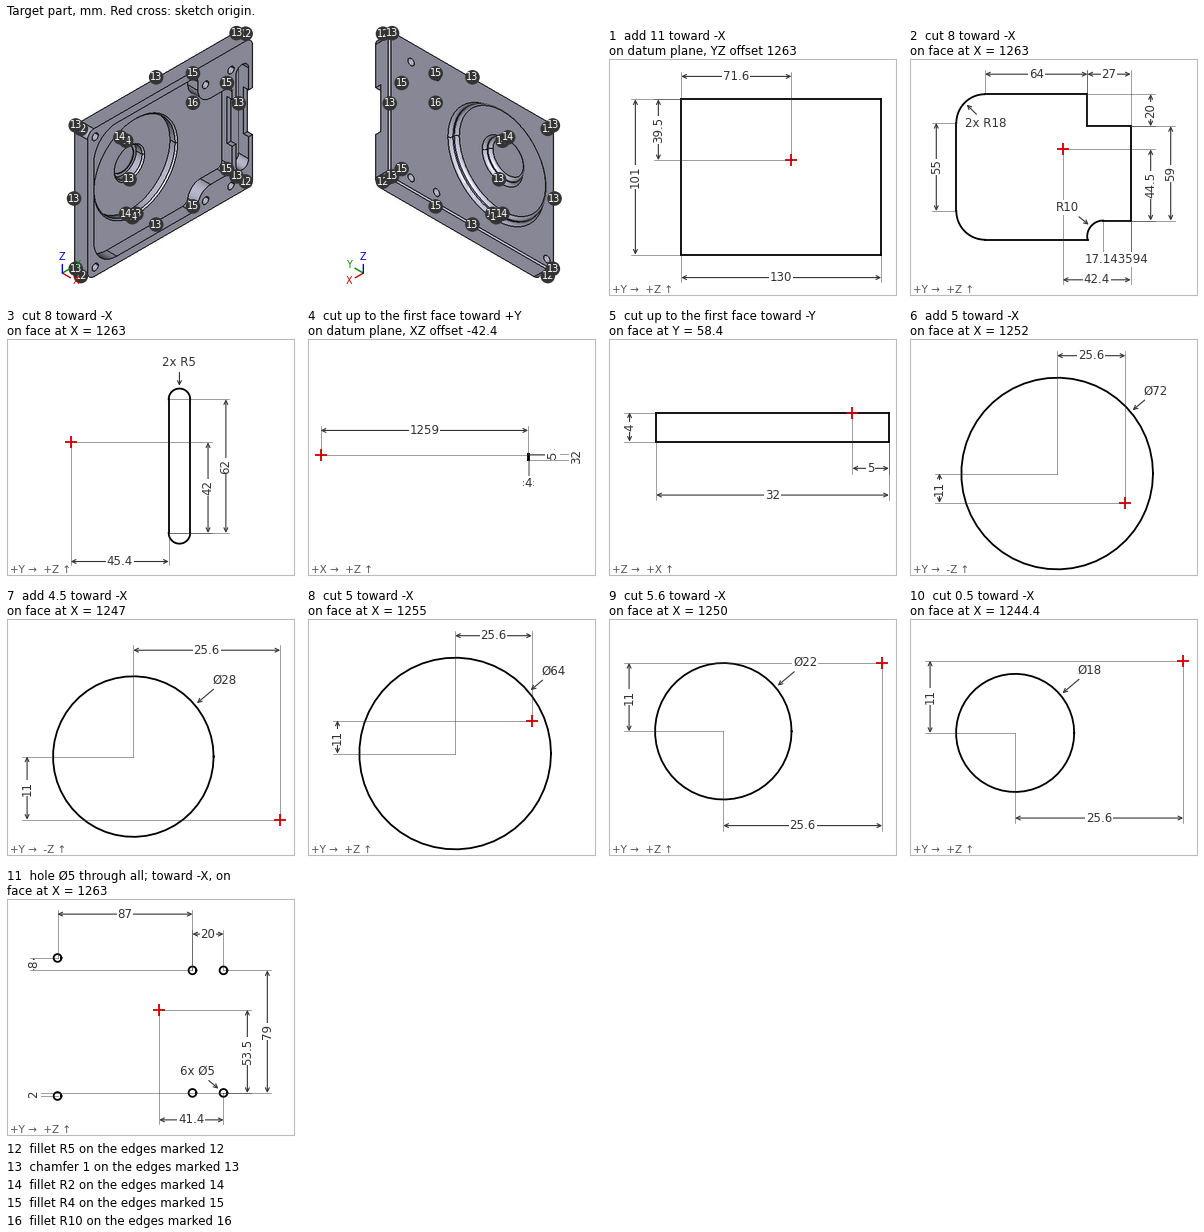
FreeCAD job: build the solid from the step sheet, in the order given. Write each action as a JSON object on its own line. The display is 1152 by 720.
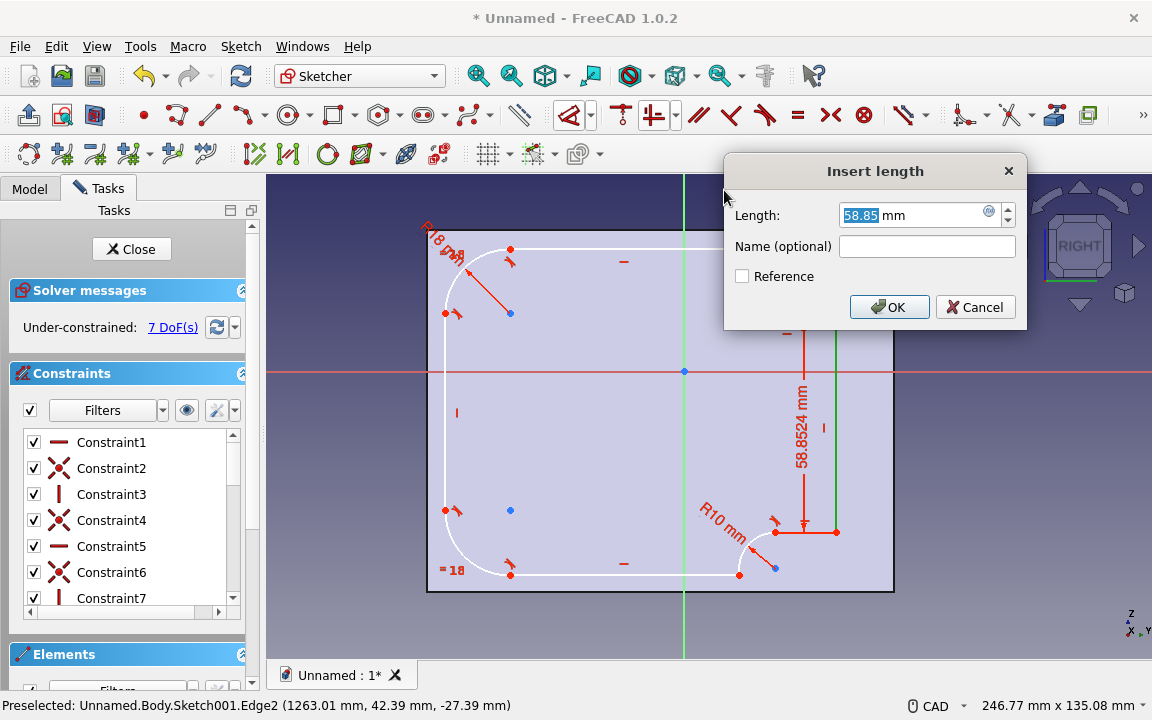
{"action": "type", "text": "59"}
{"action": "key", "text": "Return"}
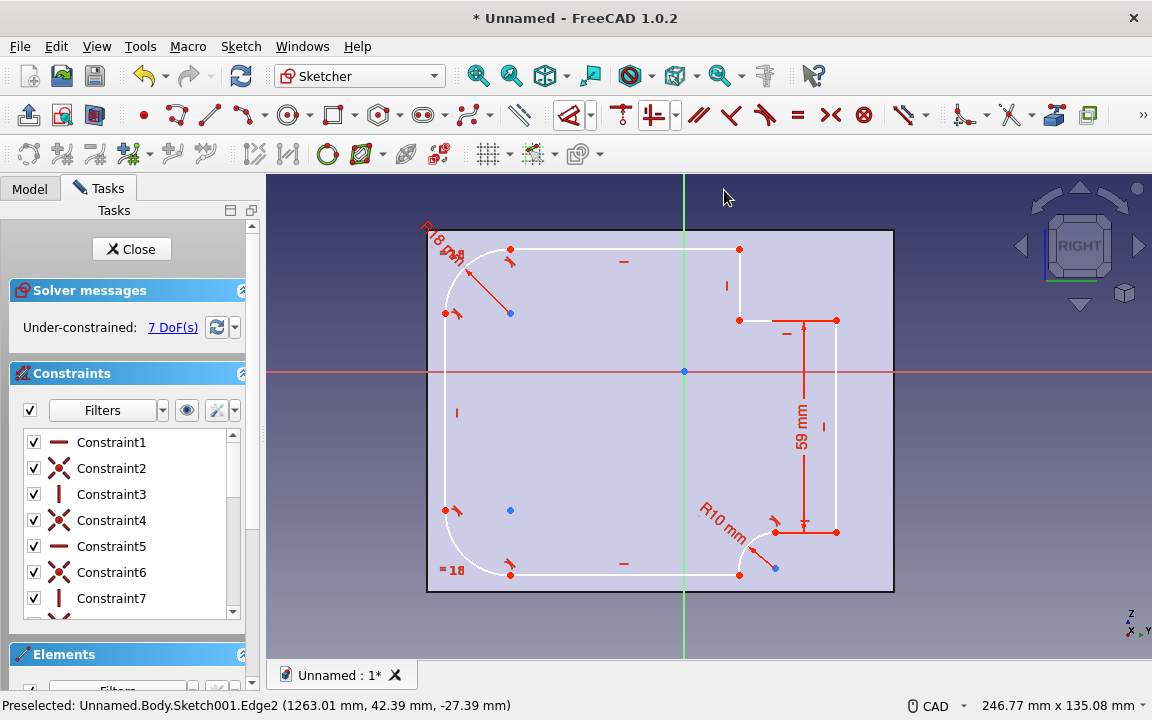
{"action": "left_click", "coordinate": [807, 321]}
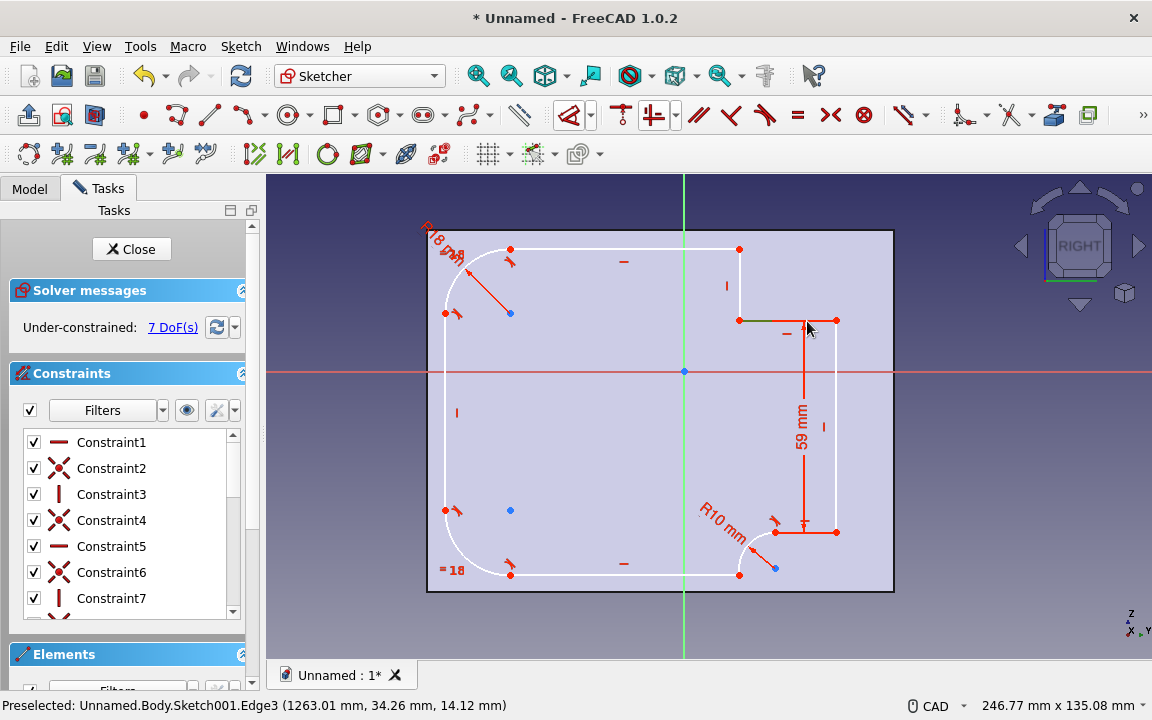
{"action": "key", "text": "l"}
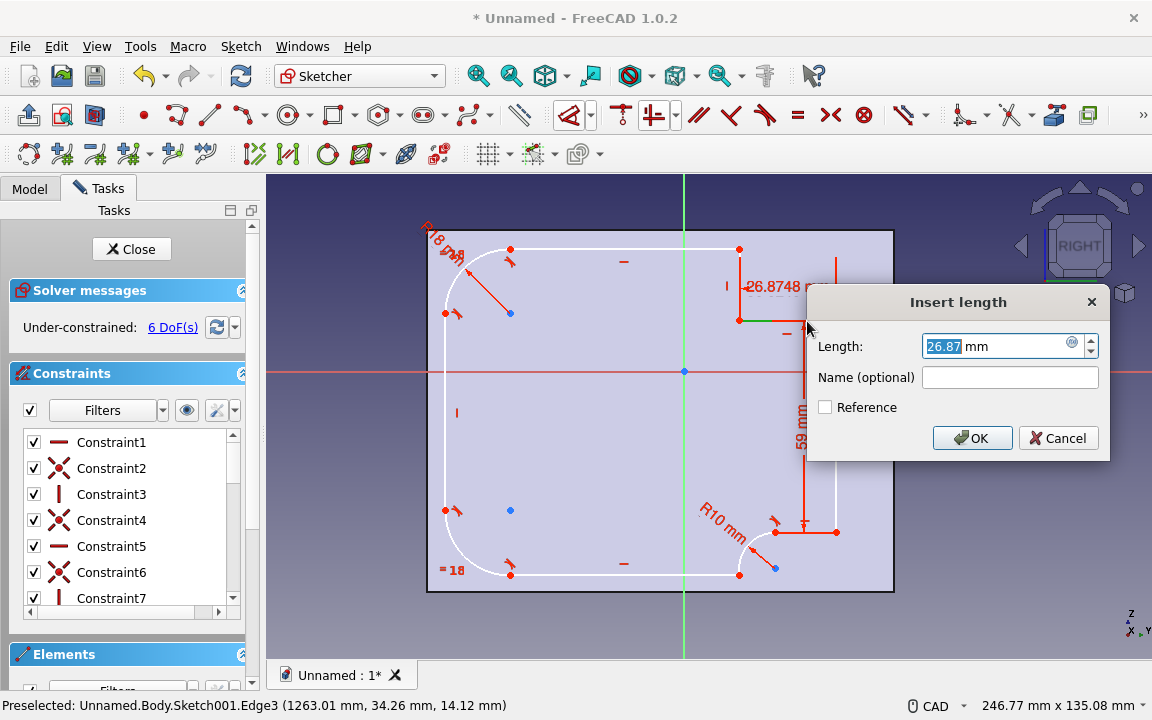
{"action": "type", "text": "27"}
{"action": "key", "text": "Return"}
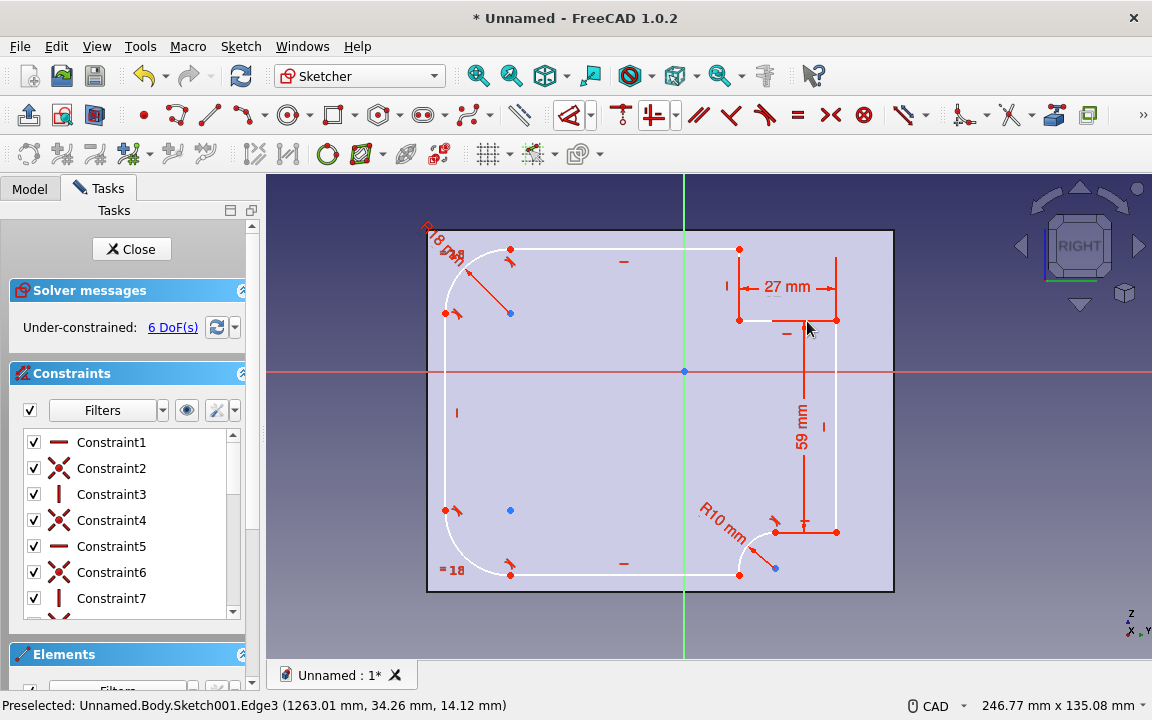
{"action": "left_click", "coordinate": [739, 299]}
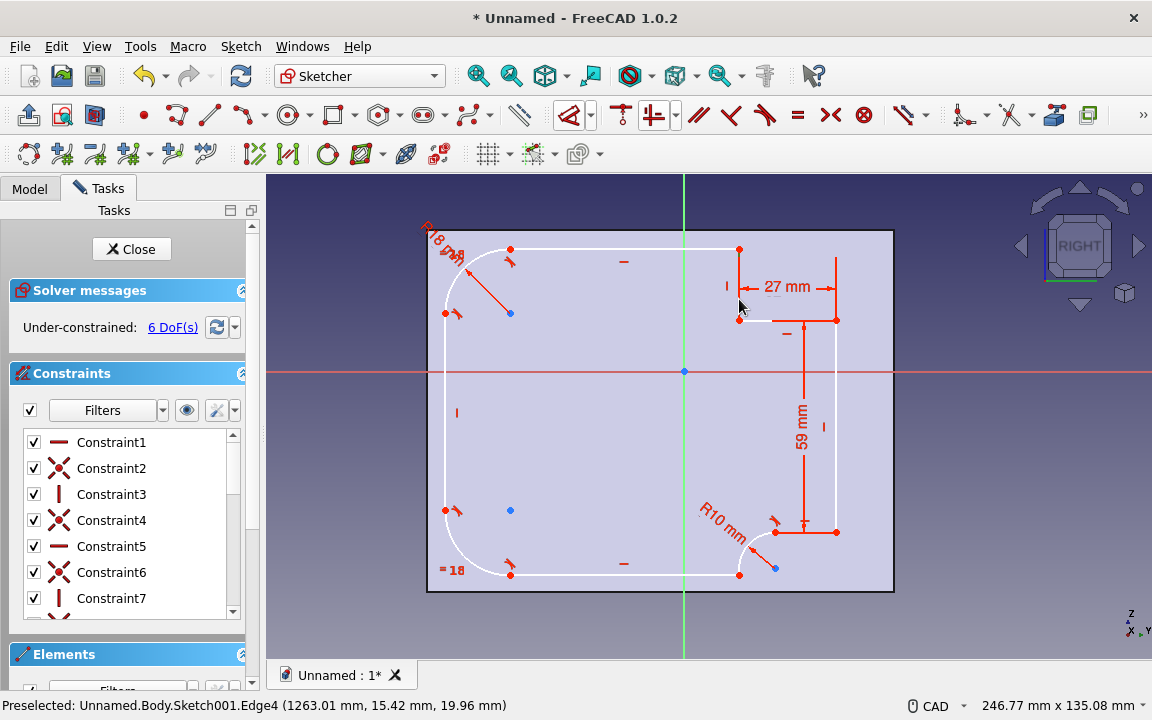
{"action": "left_click", "coordinate": [590, 116]}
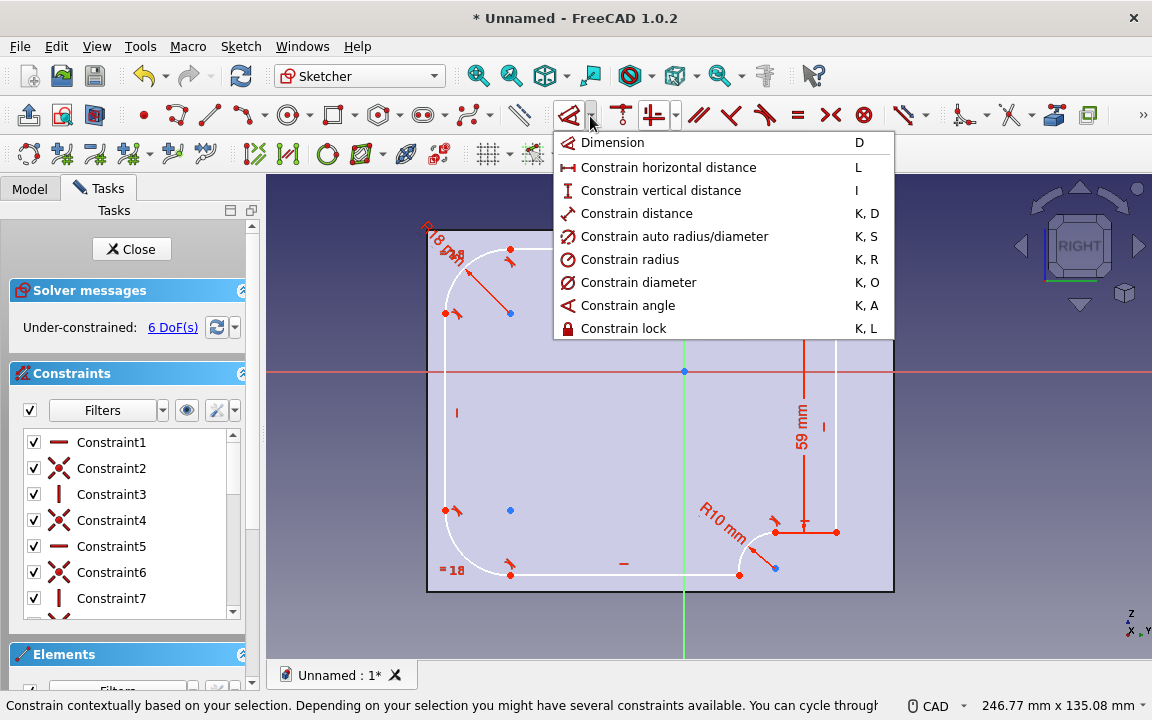
{"action": "left_click", "coordinate": [724, 190]}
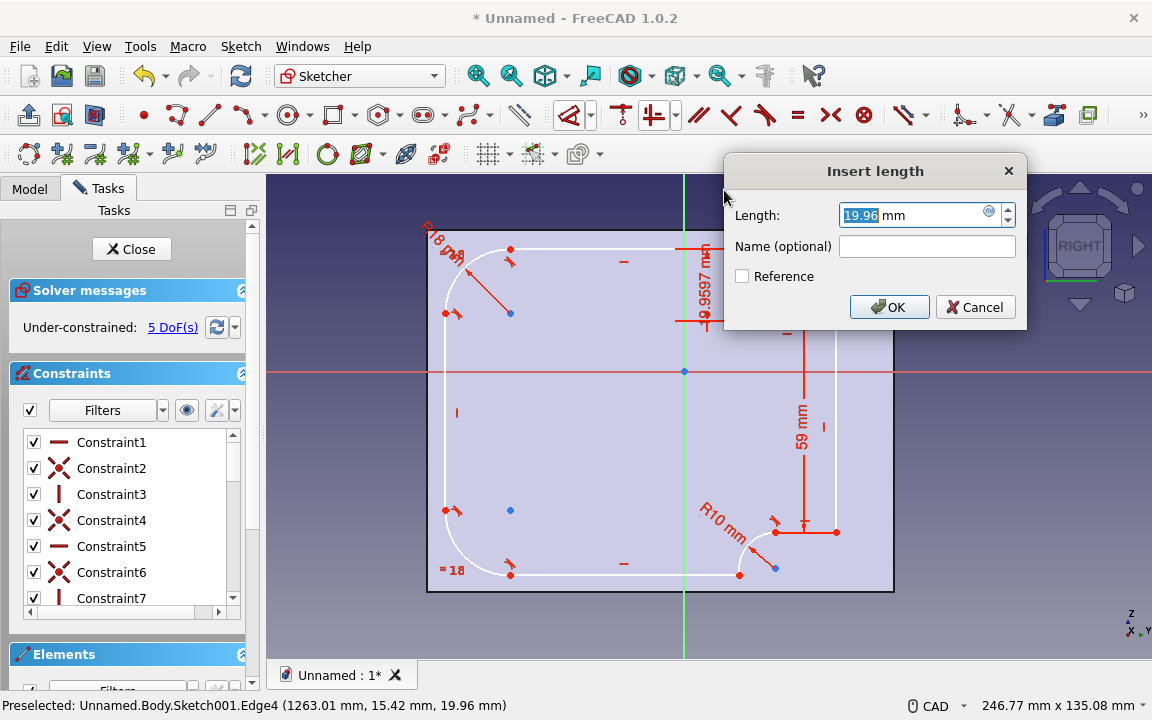
{"action": "type", "text": "20"}
{"action": "key", "text": "Return"}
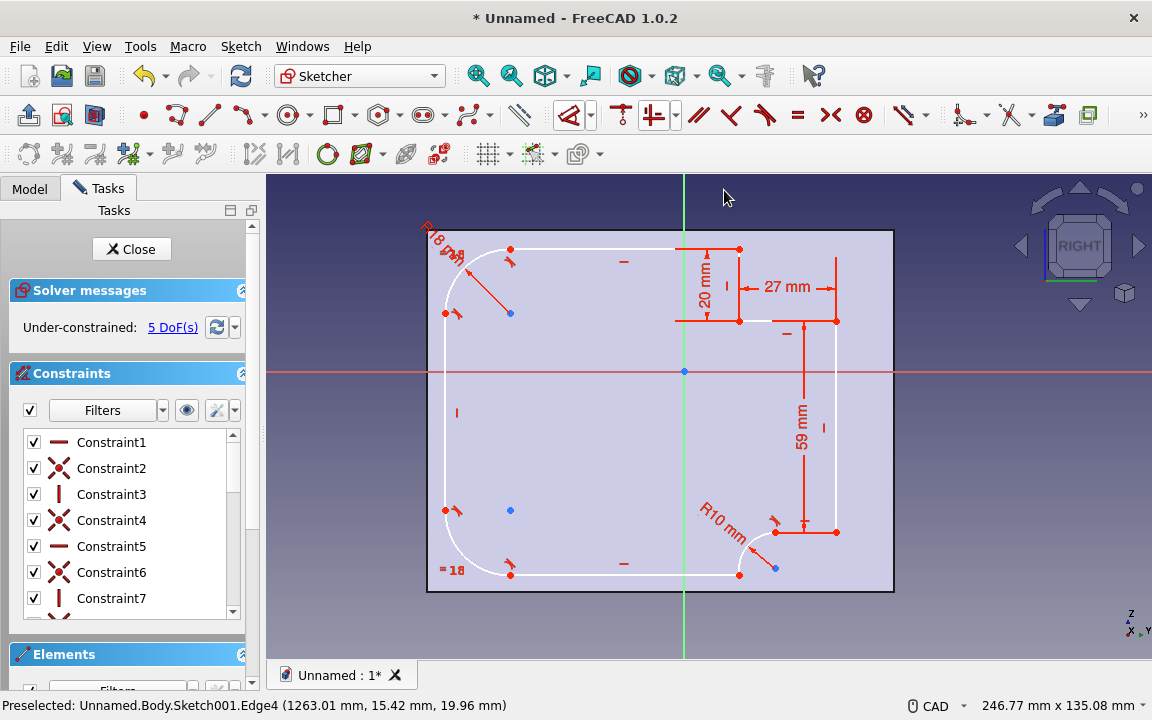
{"action": "left_click", "coordinate": [671, 249]}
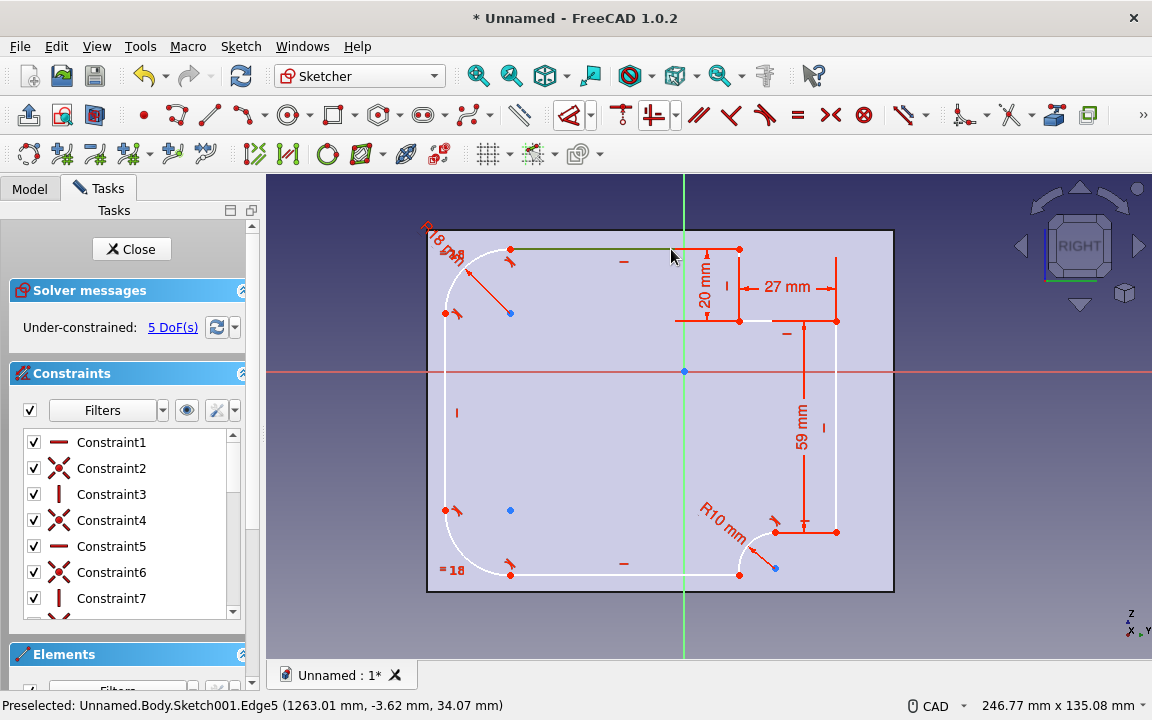
{"action": "key", "text": "l"}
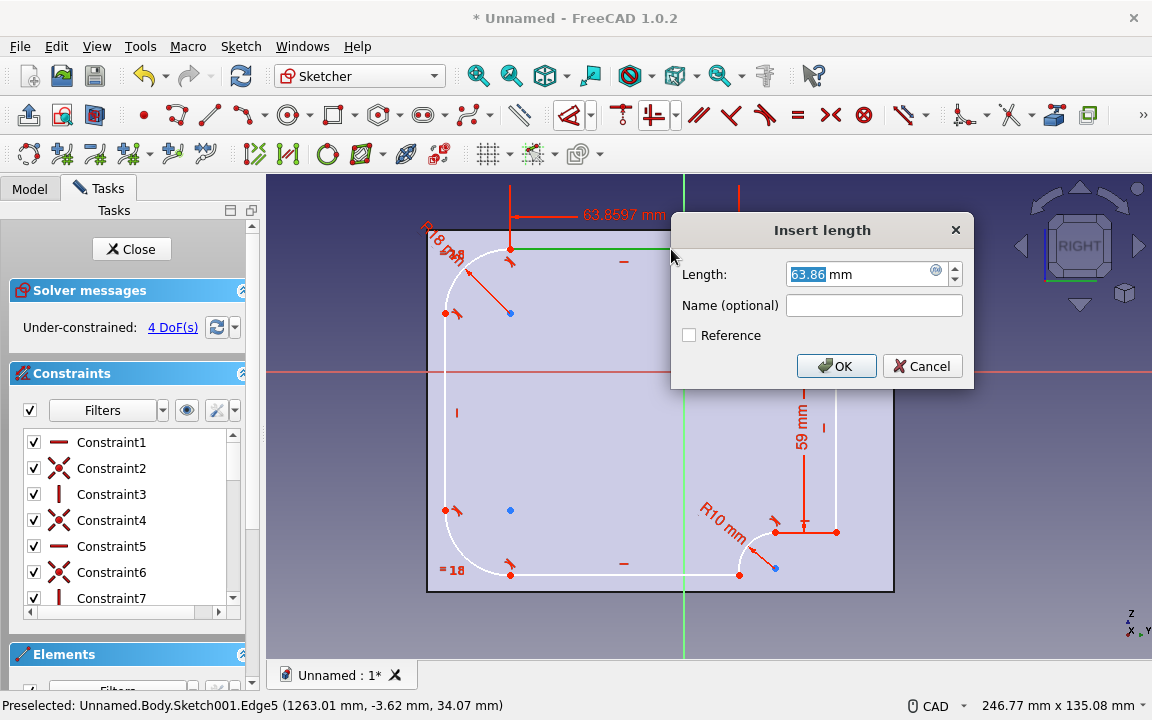
{"action": "type", "text": "64"}
{"action": "key", "text": "Return"}